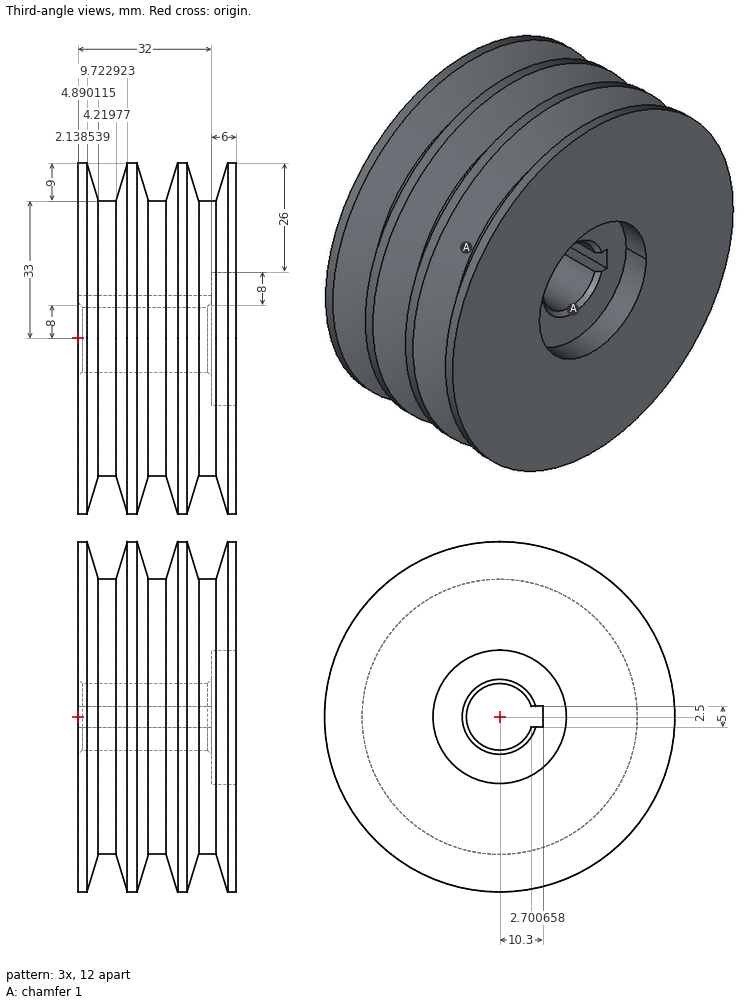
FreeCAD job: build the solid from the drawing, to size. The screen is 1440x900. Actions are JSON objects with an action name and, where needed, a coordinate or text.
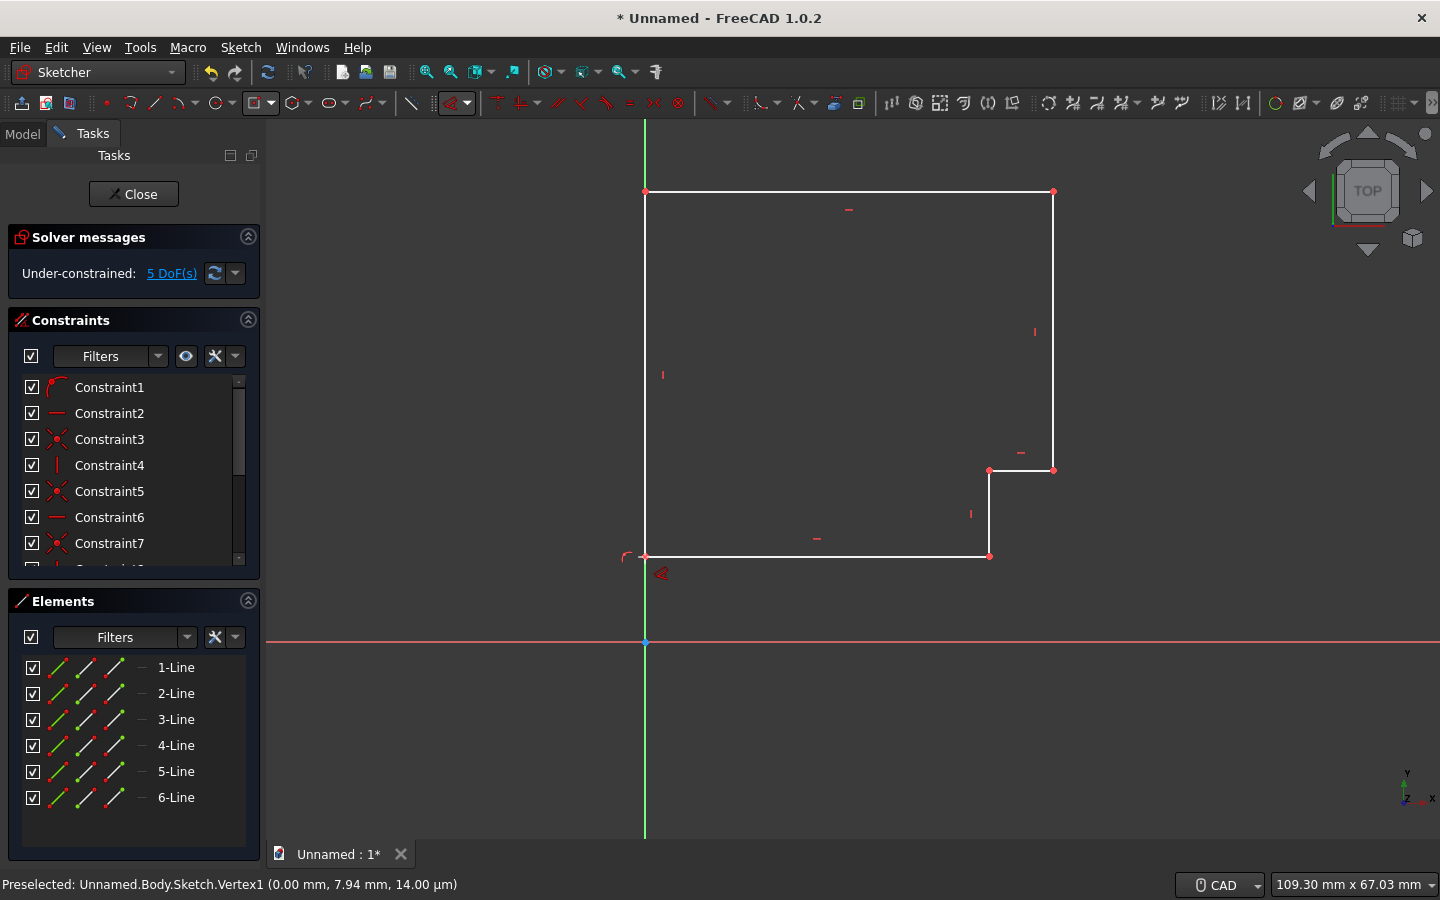
{"action": "left_click", "coordinate": [989, 531]}
{"action": "left_click", "coordinate": [1023, 514]}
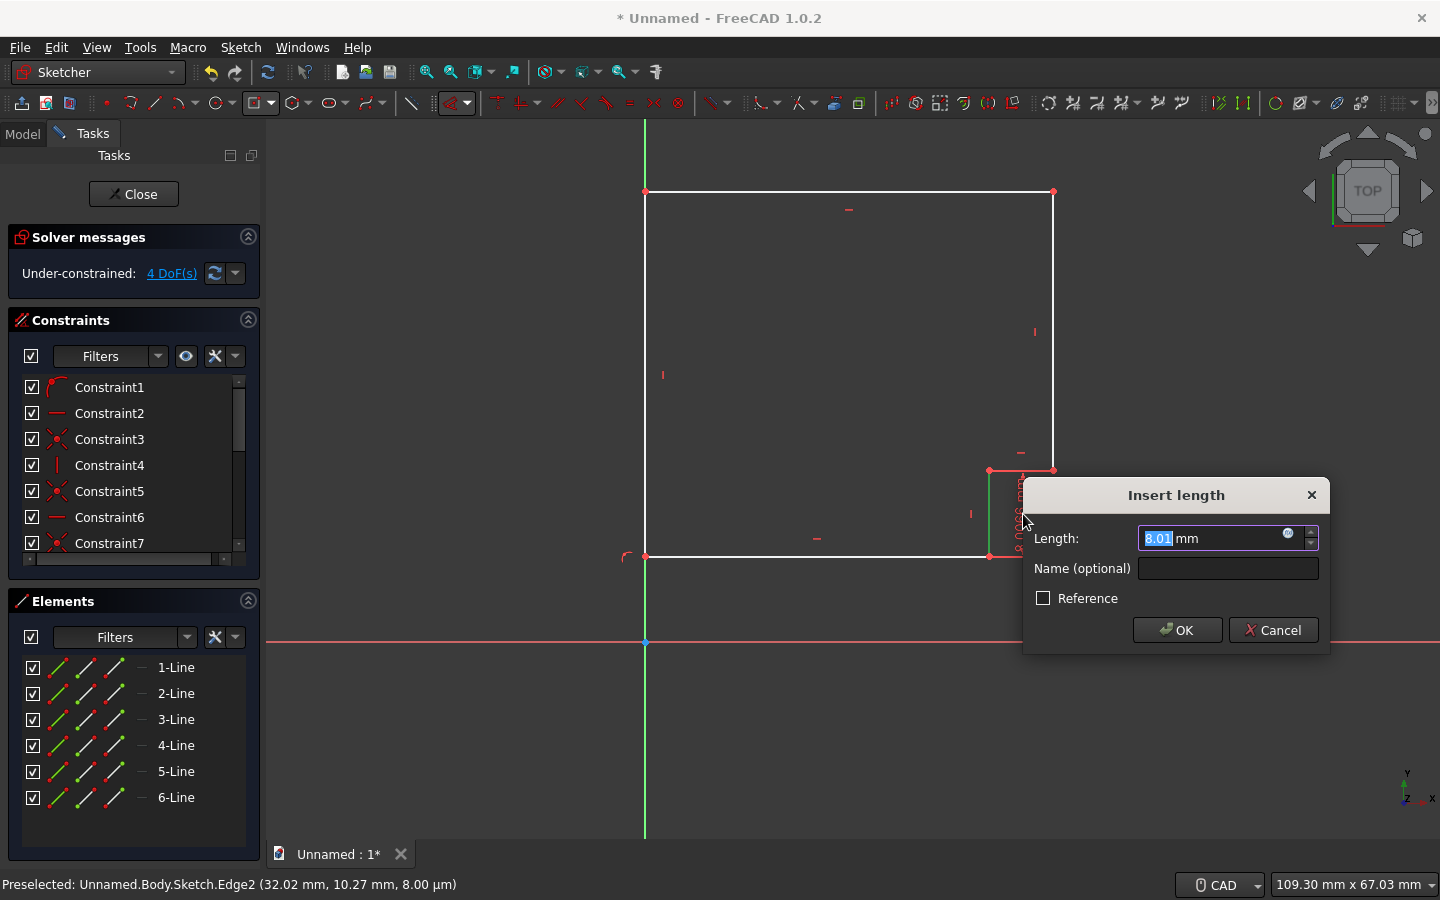
{"action": "type", "text": "8"}
{"action": "key", "text": "Return"}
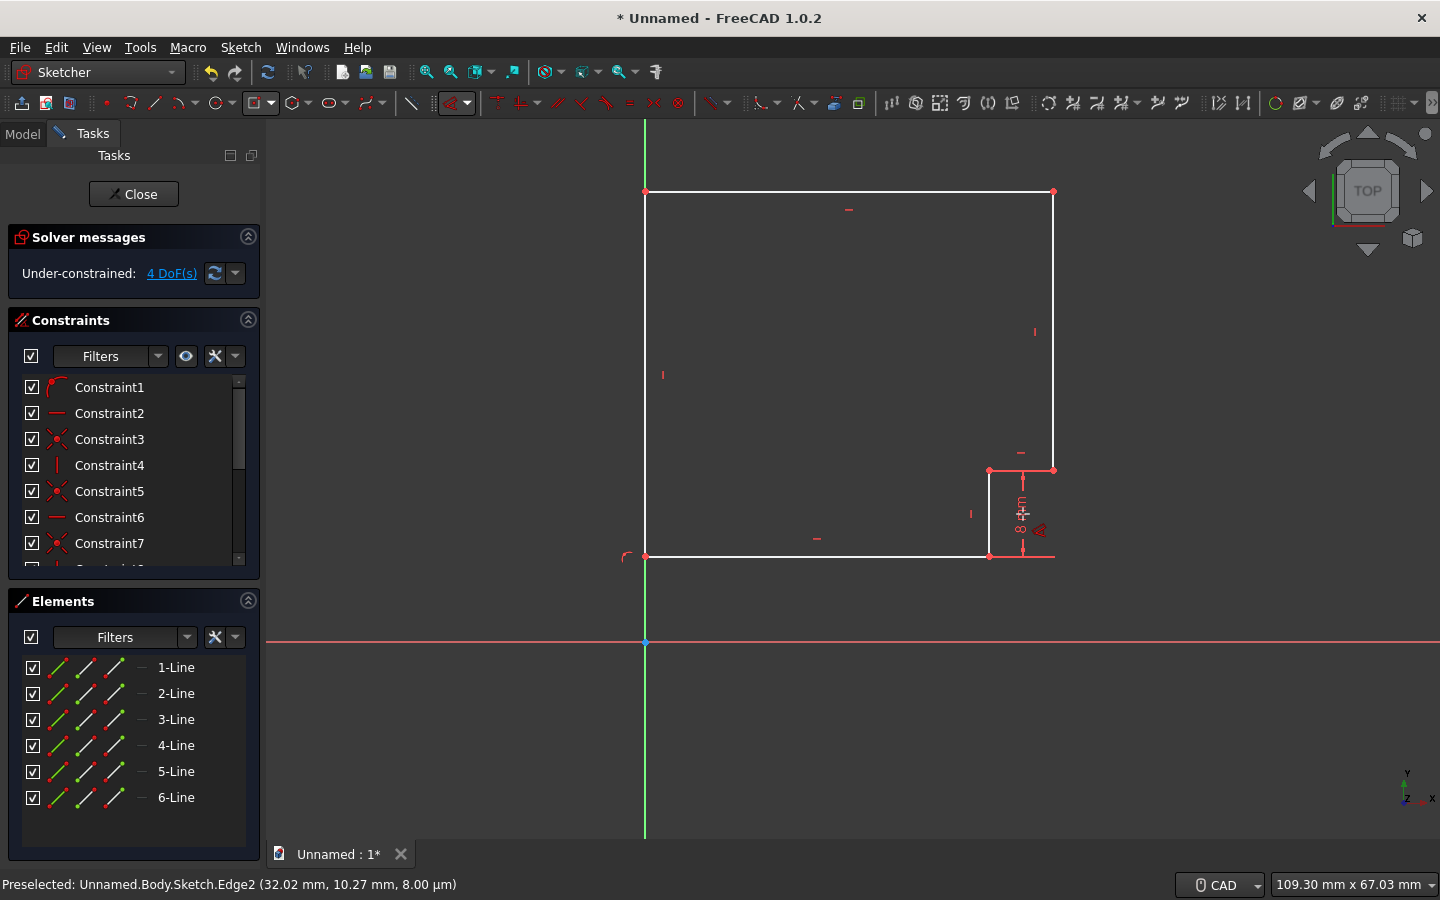
{"action": "left_click", "coordinate": [1008, 471]}
{"action": "left_click", "coordinate": [1021, 437]}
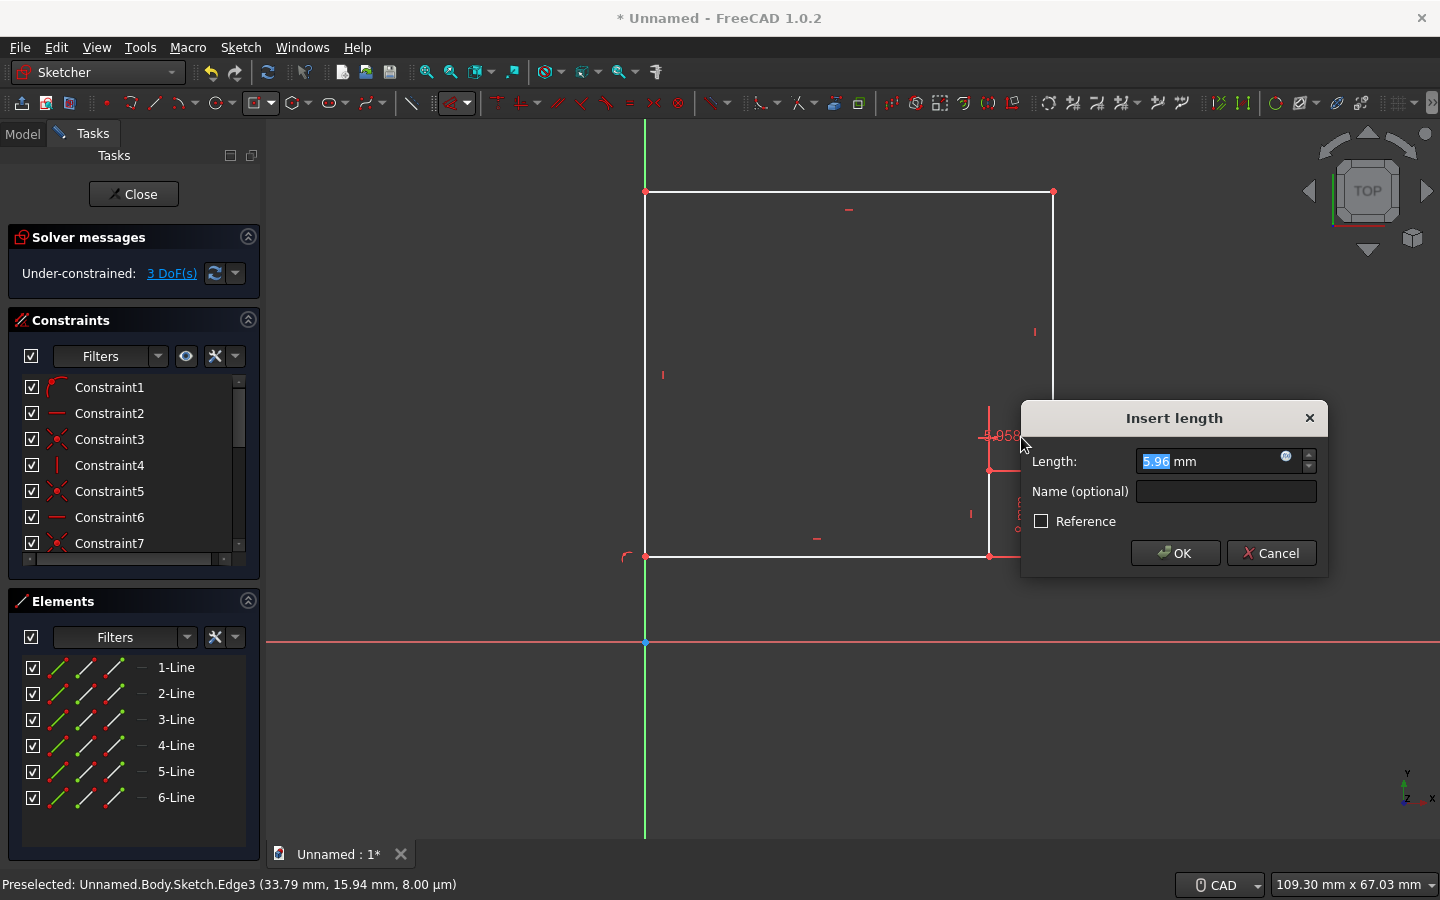
{"action": "type", "text": "6"}
{"action": "key", "text": "Return"}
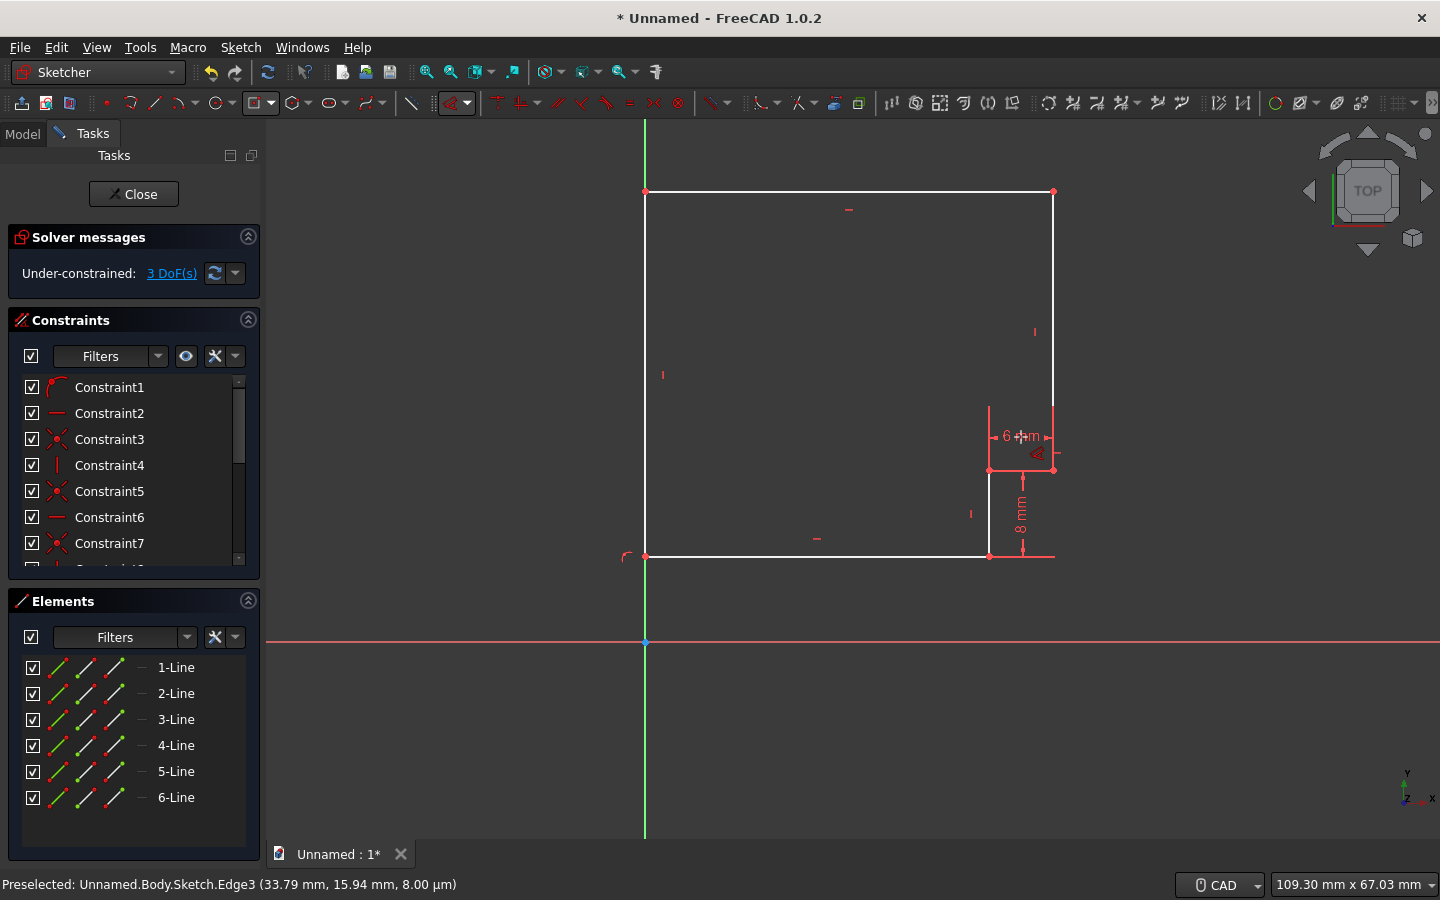
{"action": "left_click", "coordinate": [748, 557]}
{"action": "left_click", "coordinate": [817, 591]}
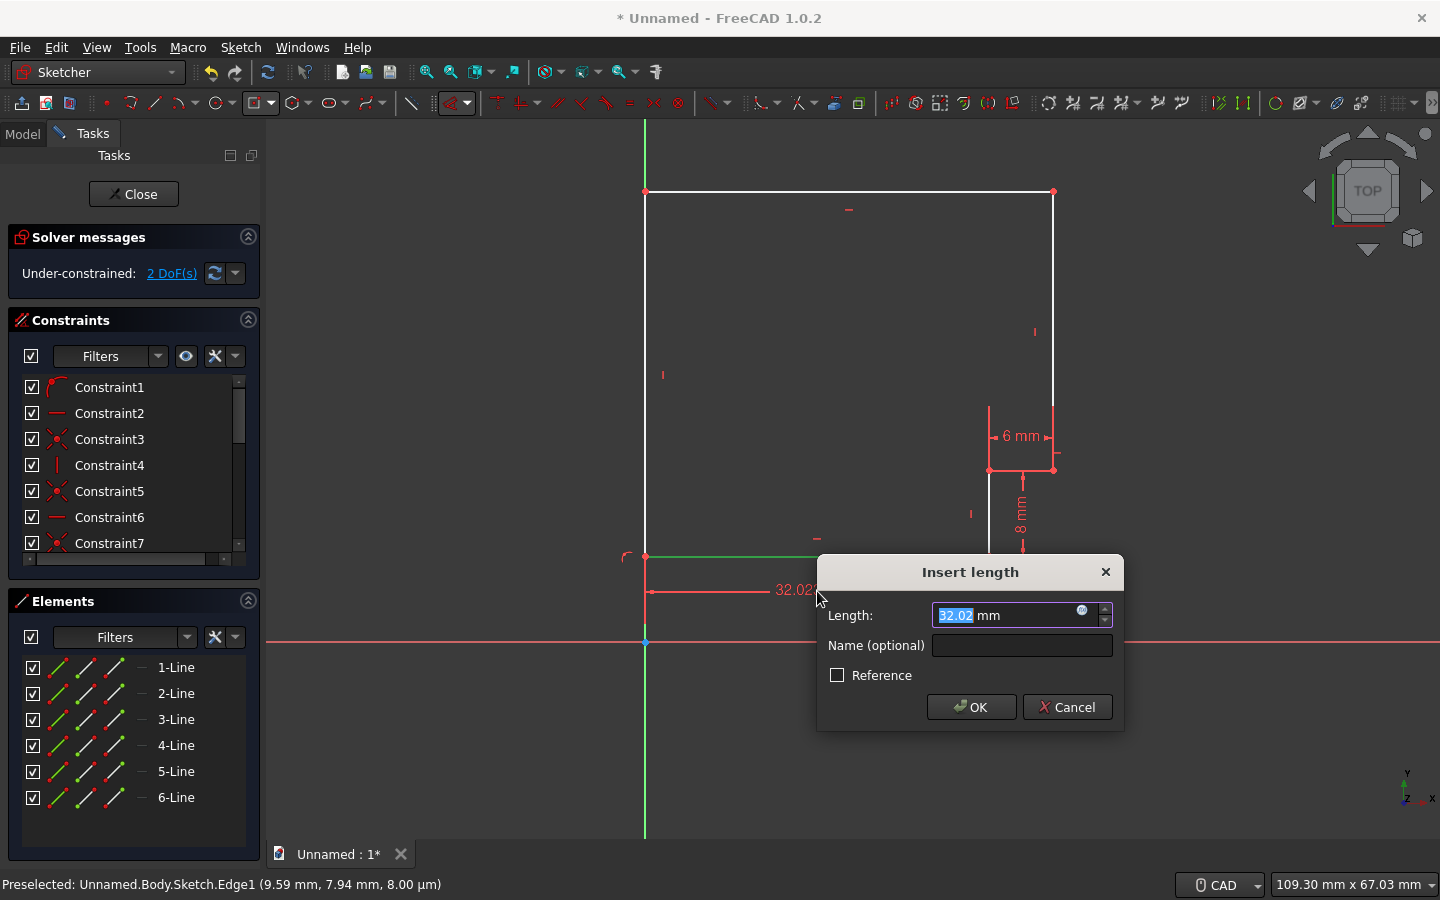
{"action": "type", "text": "32"}
{"action": "key", "text": "Return"}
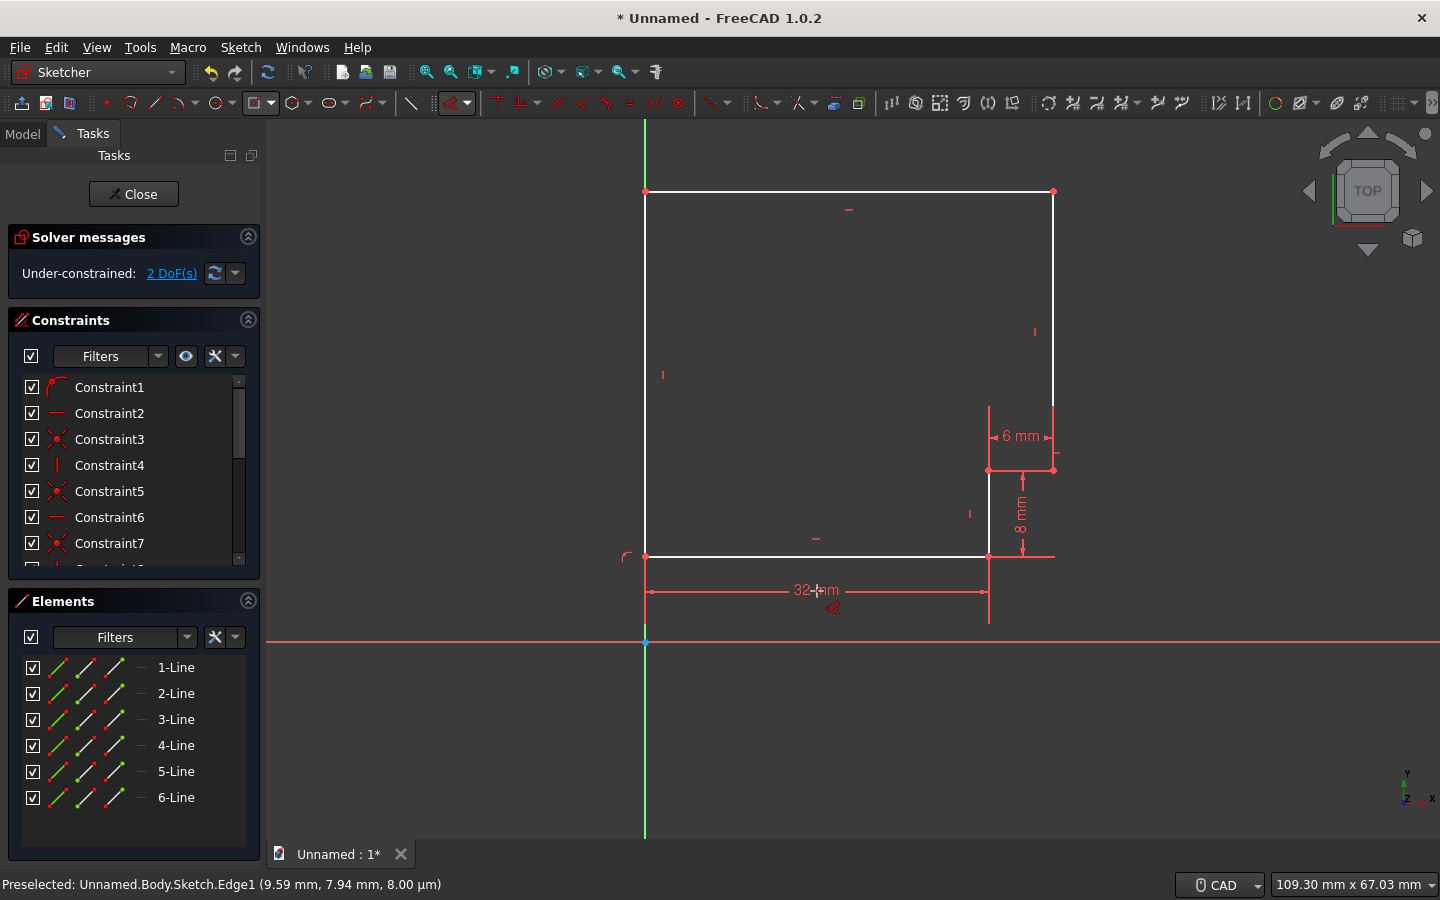
{"action": "left_click", "coordinate": [1053, 387]}
{"action": "left_click", "coordinate": [1087, 331]}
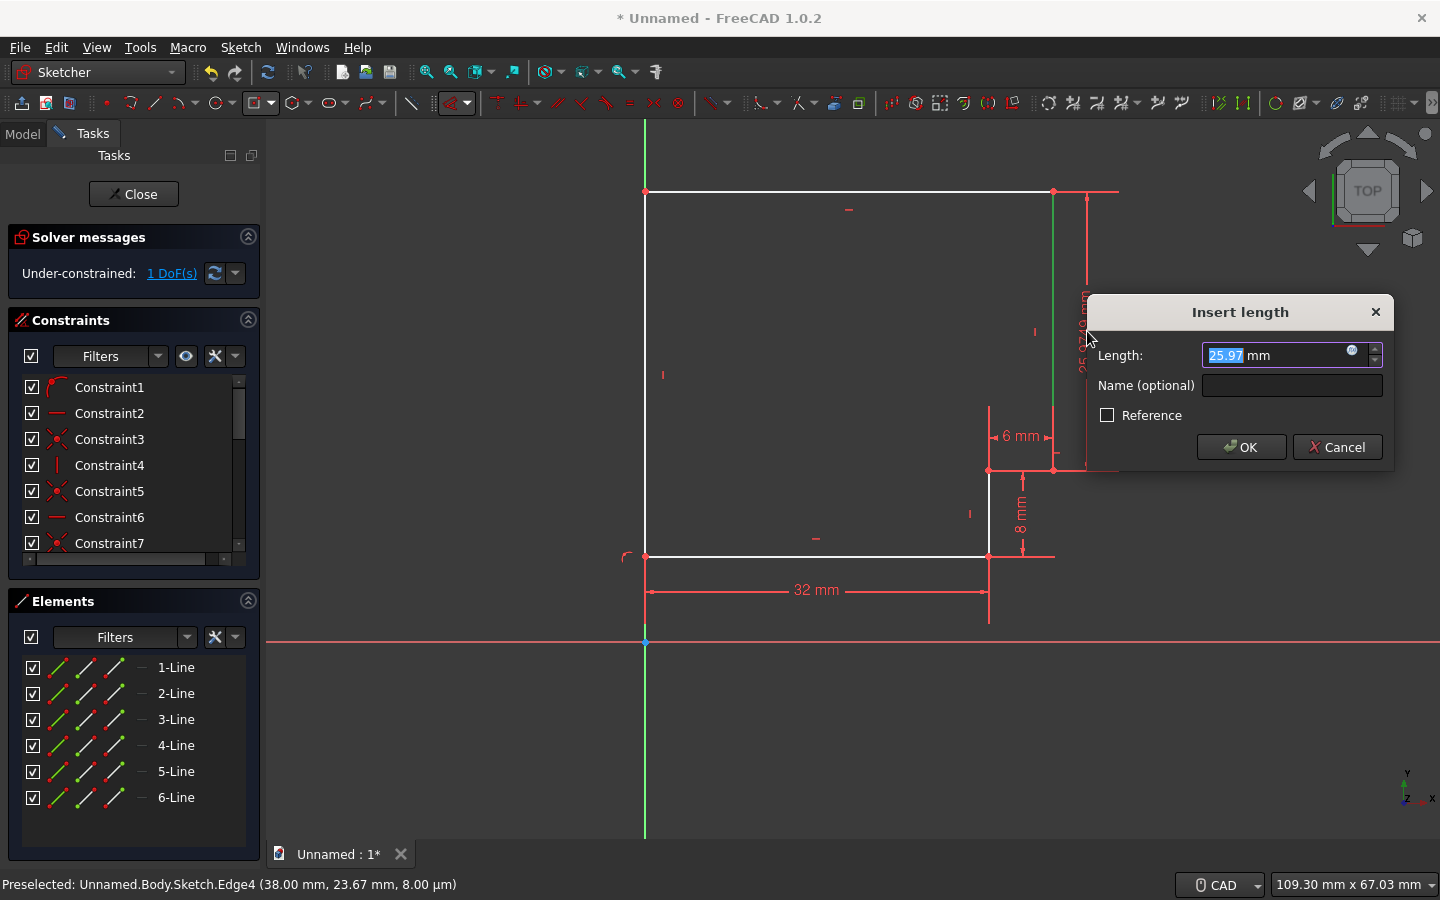
{"action": "type", "text": "26"}
{"action": "key", "text": "Return"}